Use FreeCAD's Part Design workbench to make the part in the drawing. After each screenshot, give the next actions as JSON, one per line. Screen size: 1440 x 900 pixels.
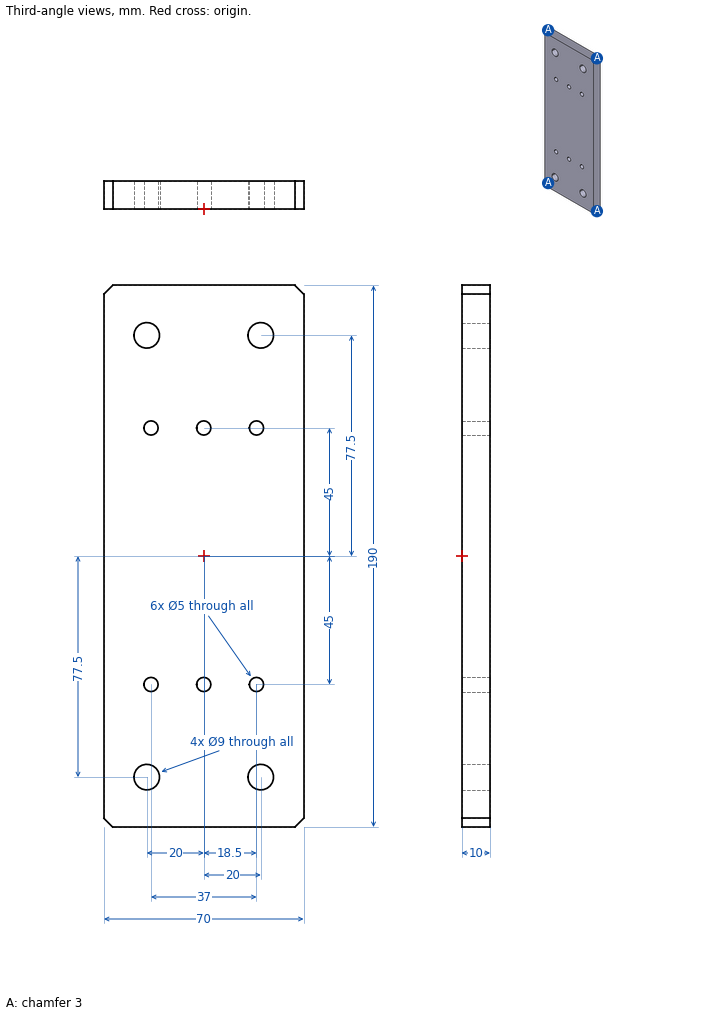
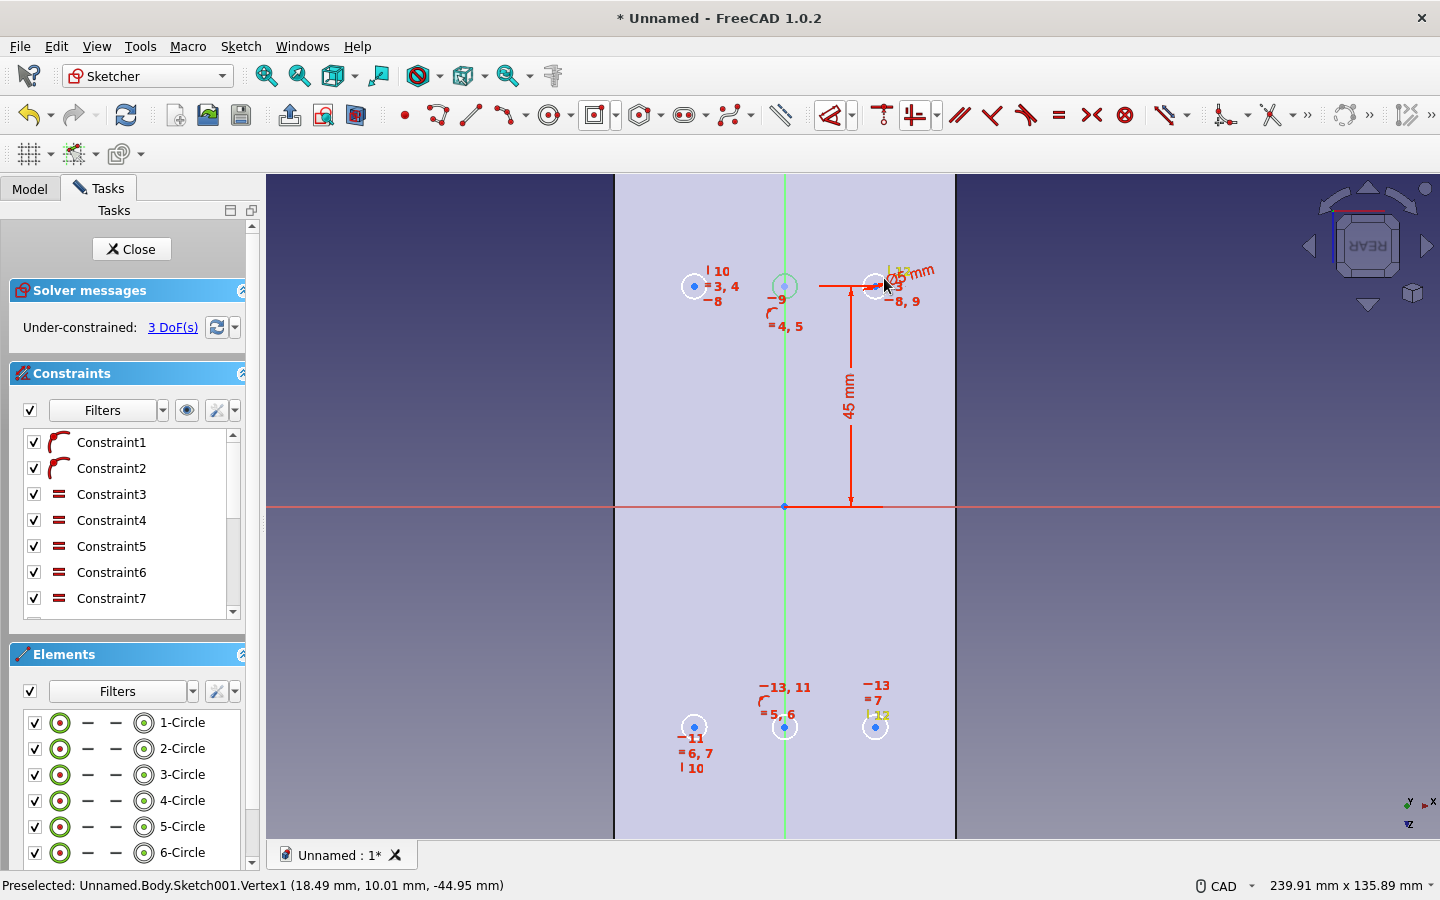
{"action": "left_click", "coordinate": [785, 727]}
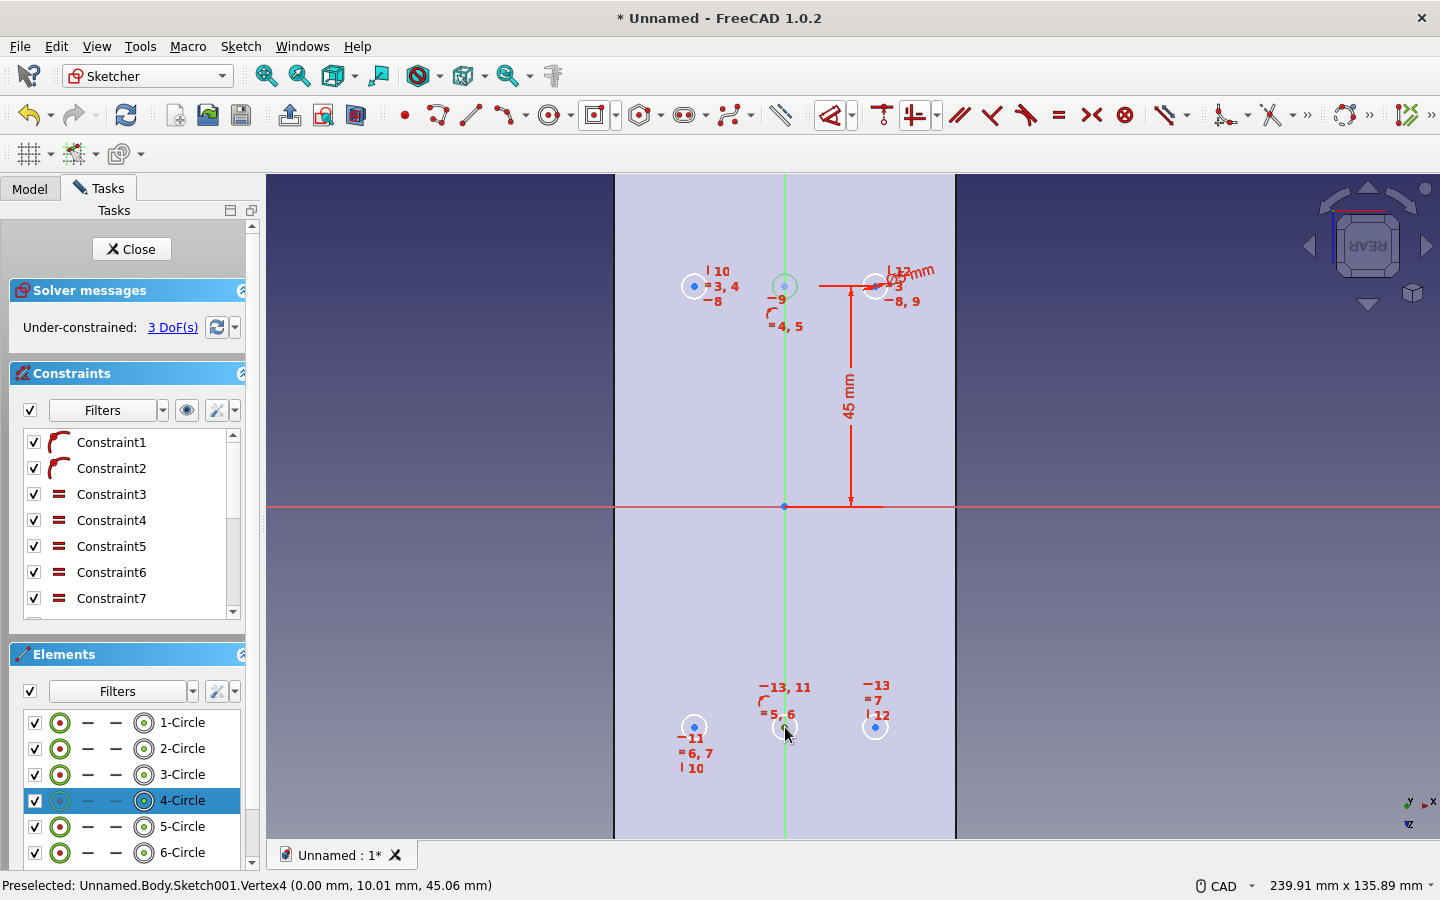
{"action": "key", "text": "i"}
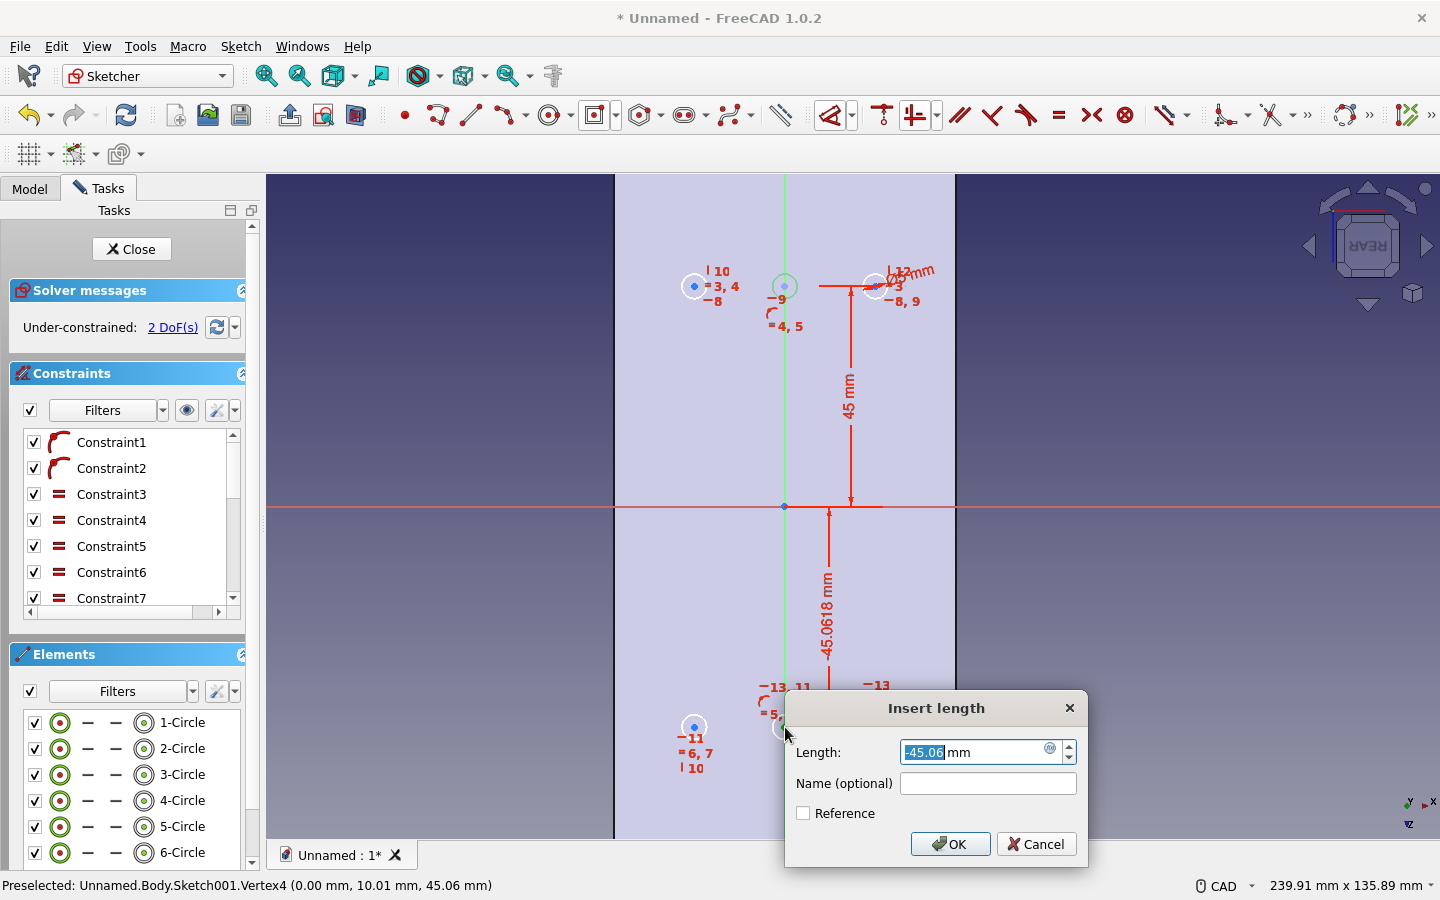
{"action": "type", "text": "-45"}
{"action": "key", "text": "Return"}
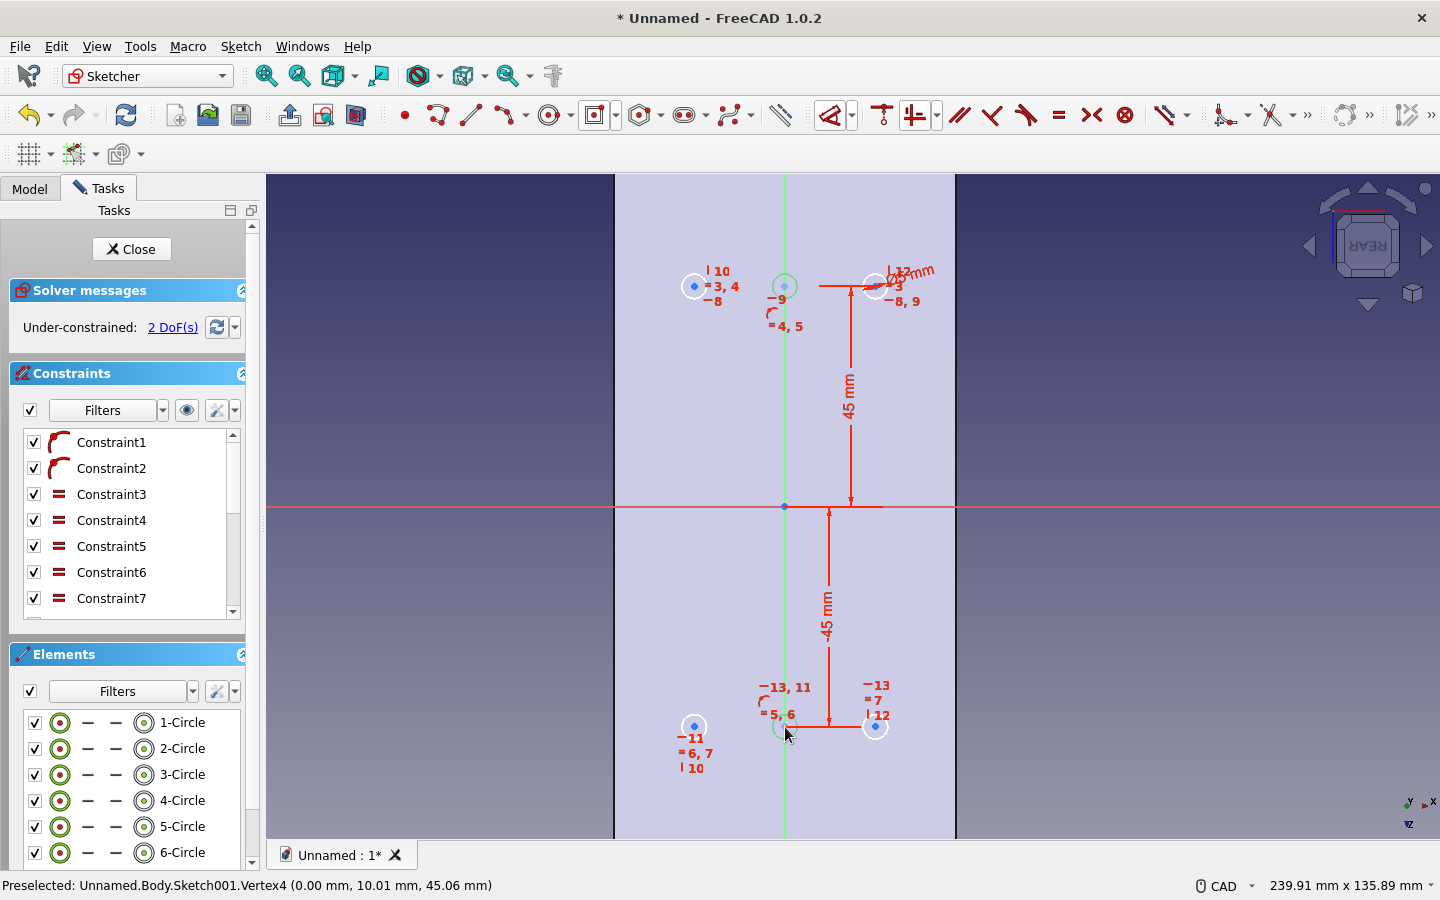
{"action": "left_click", "coordinate": [875, 286]}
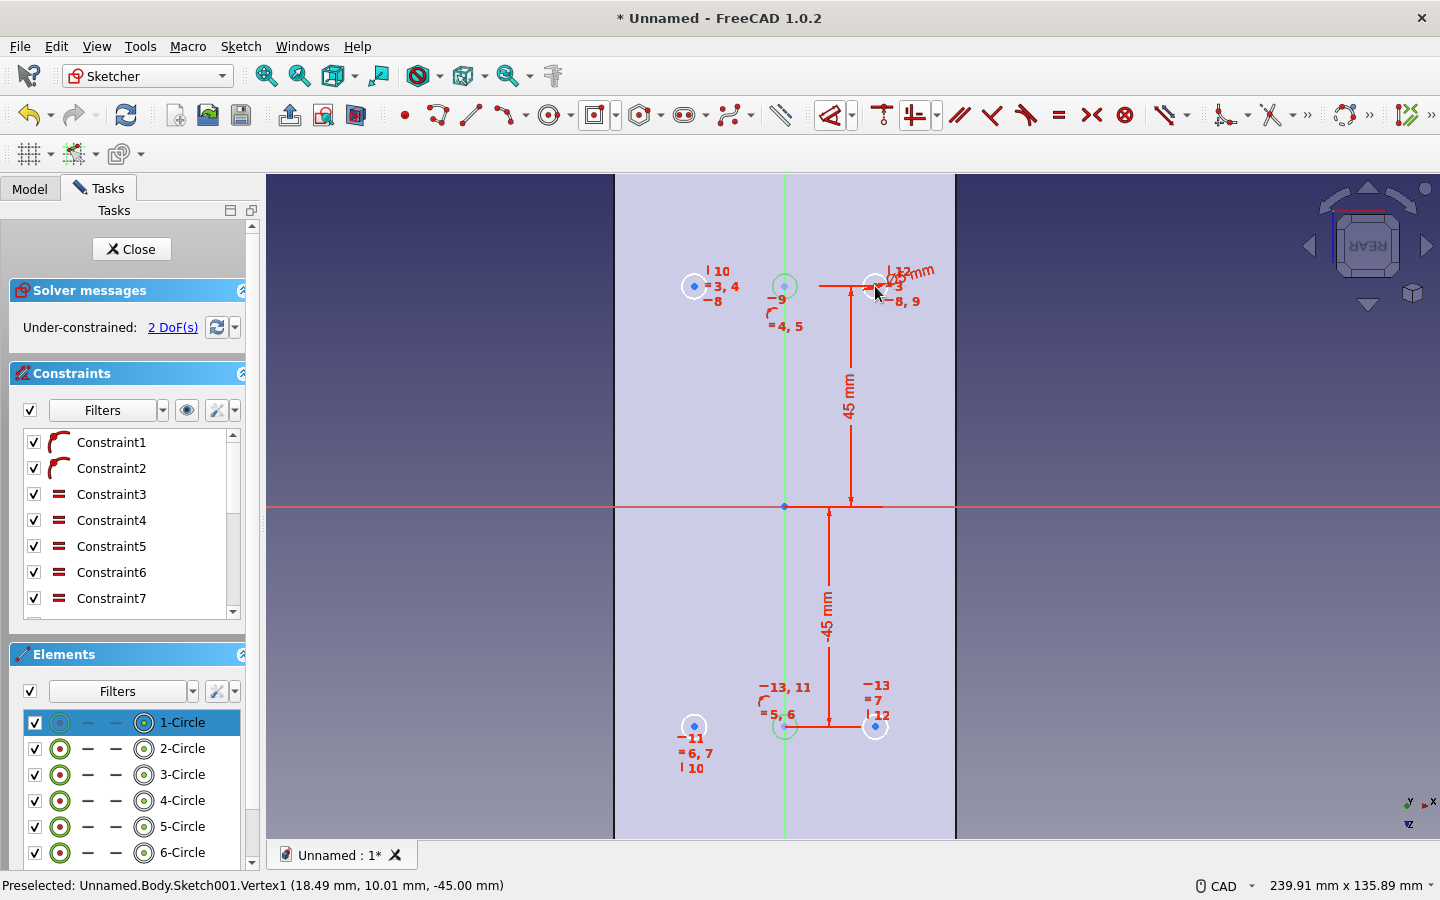
{"action": "left_click", "coordinate": [694, 286]}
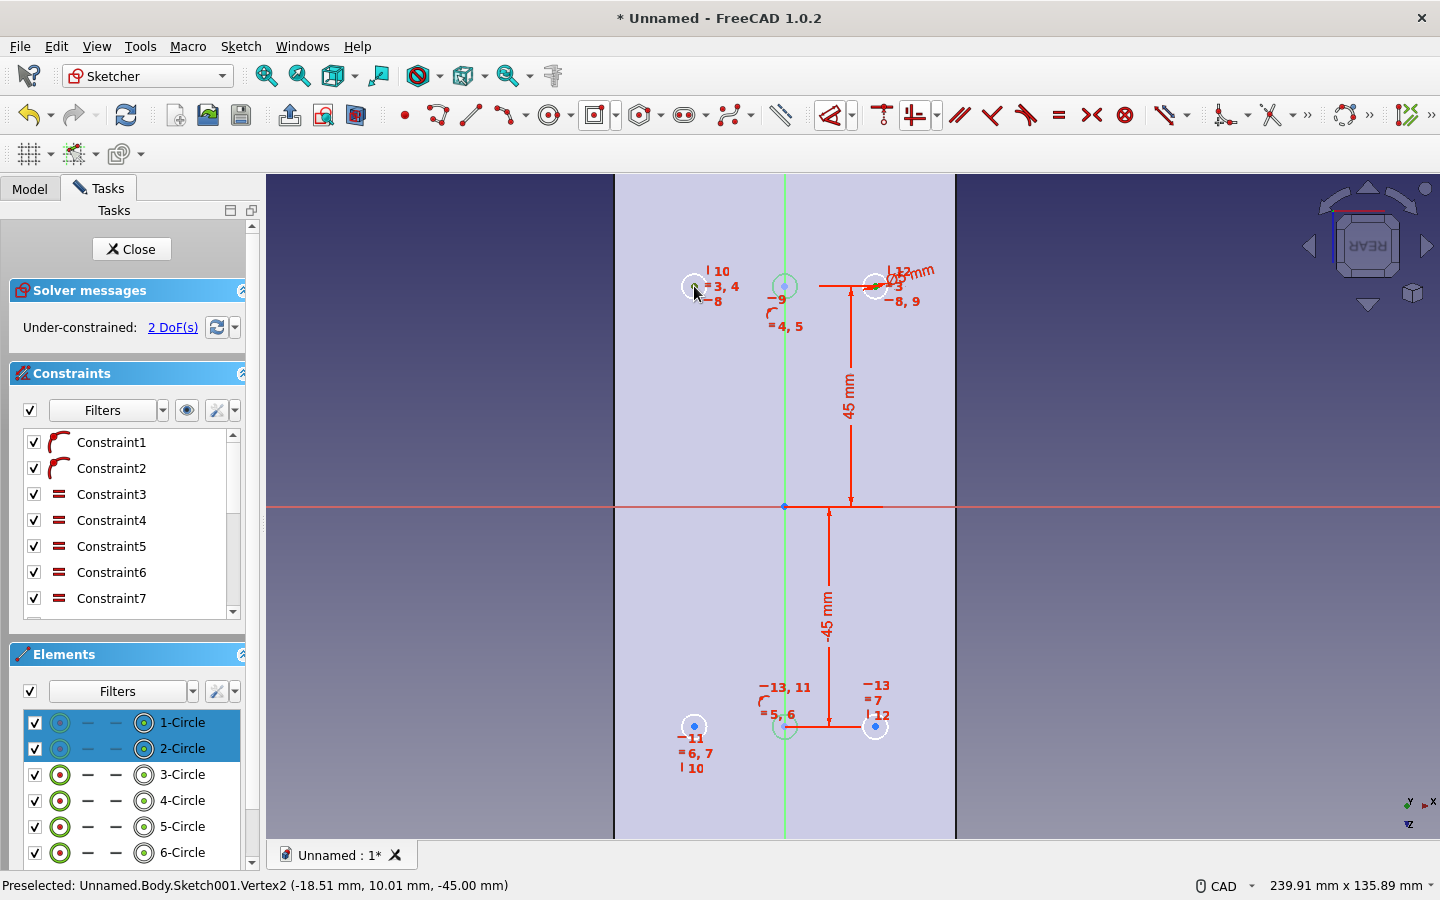
{"action": "left_click", "coordinate": [852, 116]}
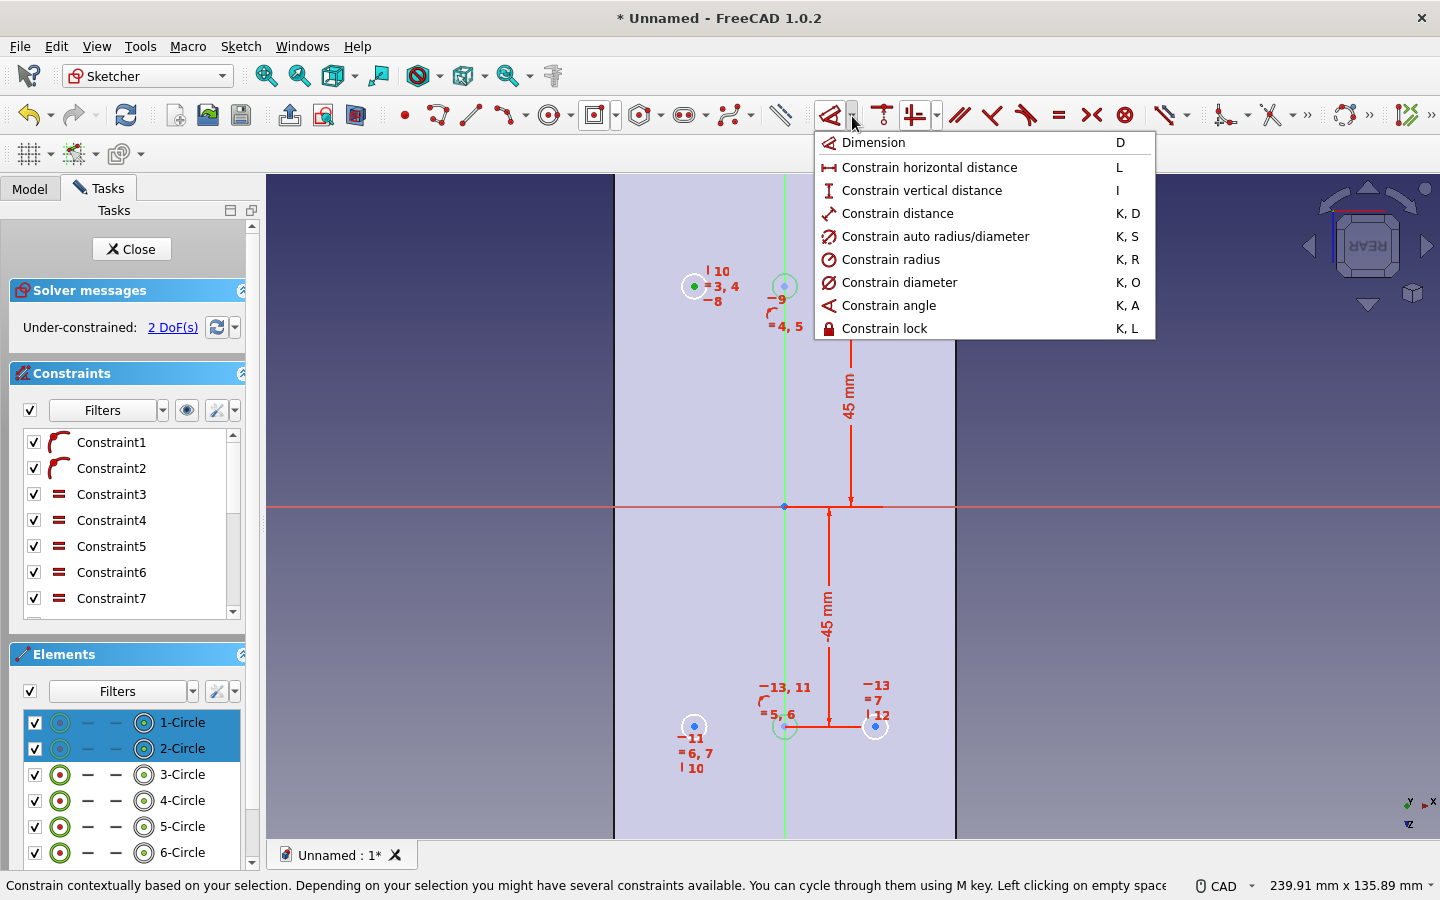
{"action": "left_click", "coordinate": [985, 168]}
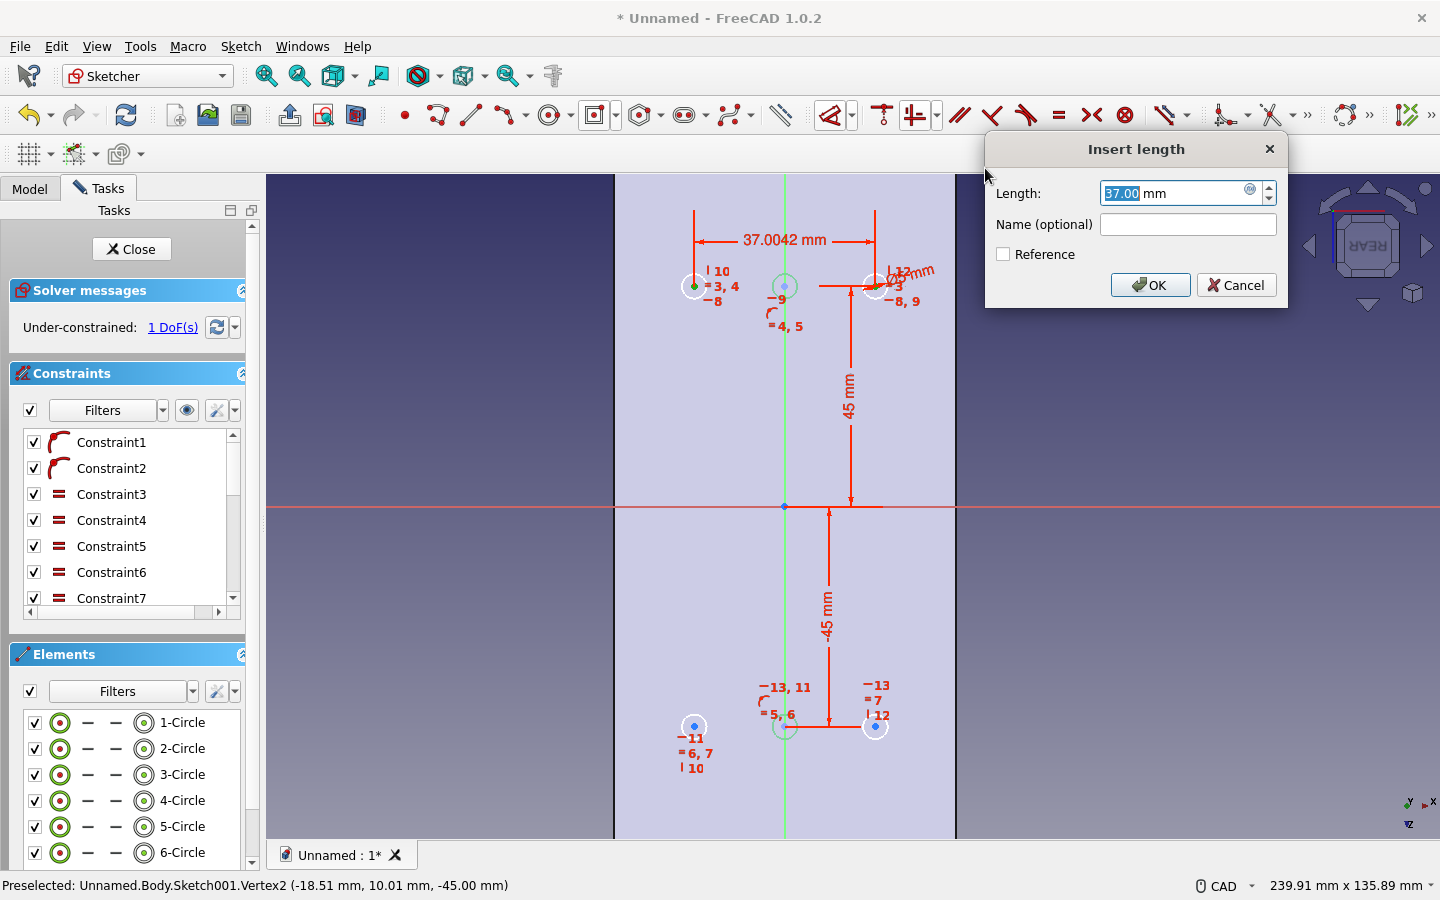
{"action": "type", "text": "37"}
{"action": "key", "text": "Return"}